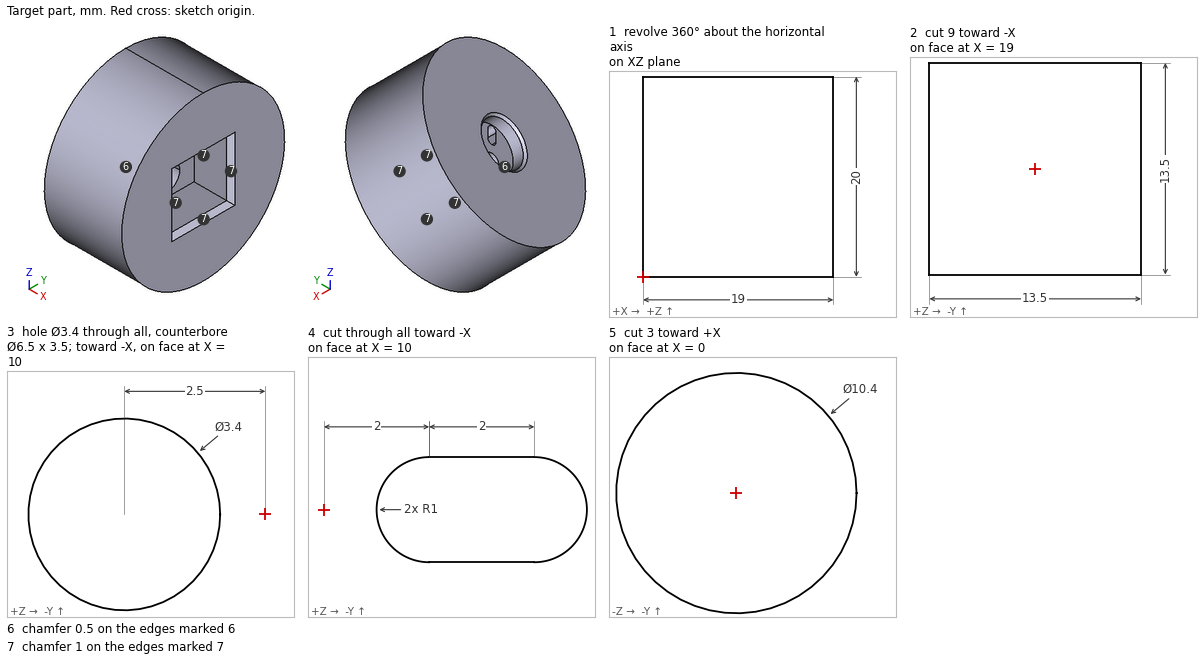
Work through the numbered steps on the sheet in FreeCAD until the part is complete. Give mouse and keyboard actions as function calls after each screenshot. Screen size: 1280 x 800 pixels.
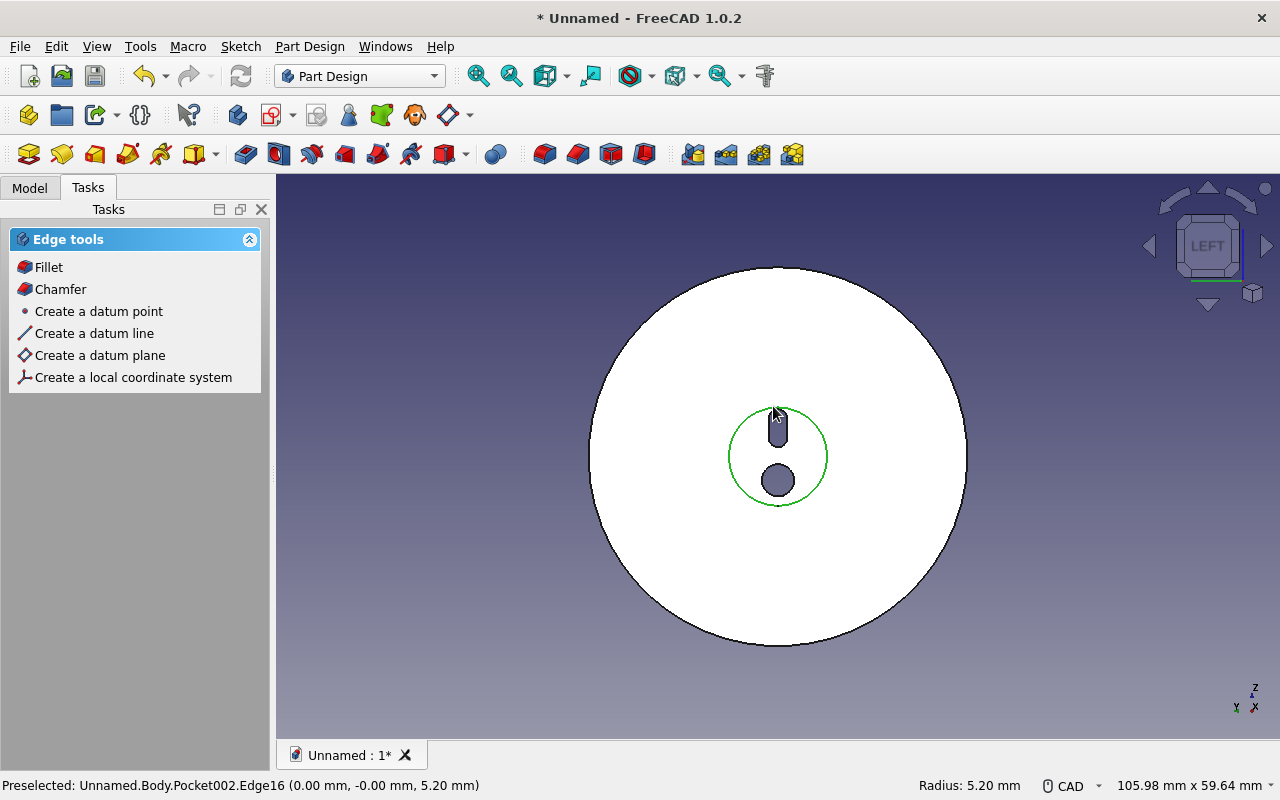
click(578, 154)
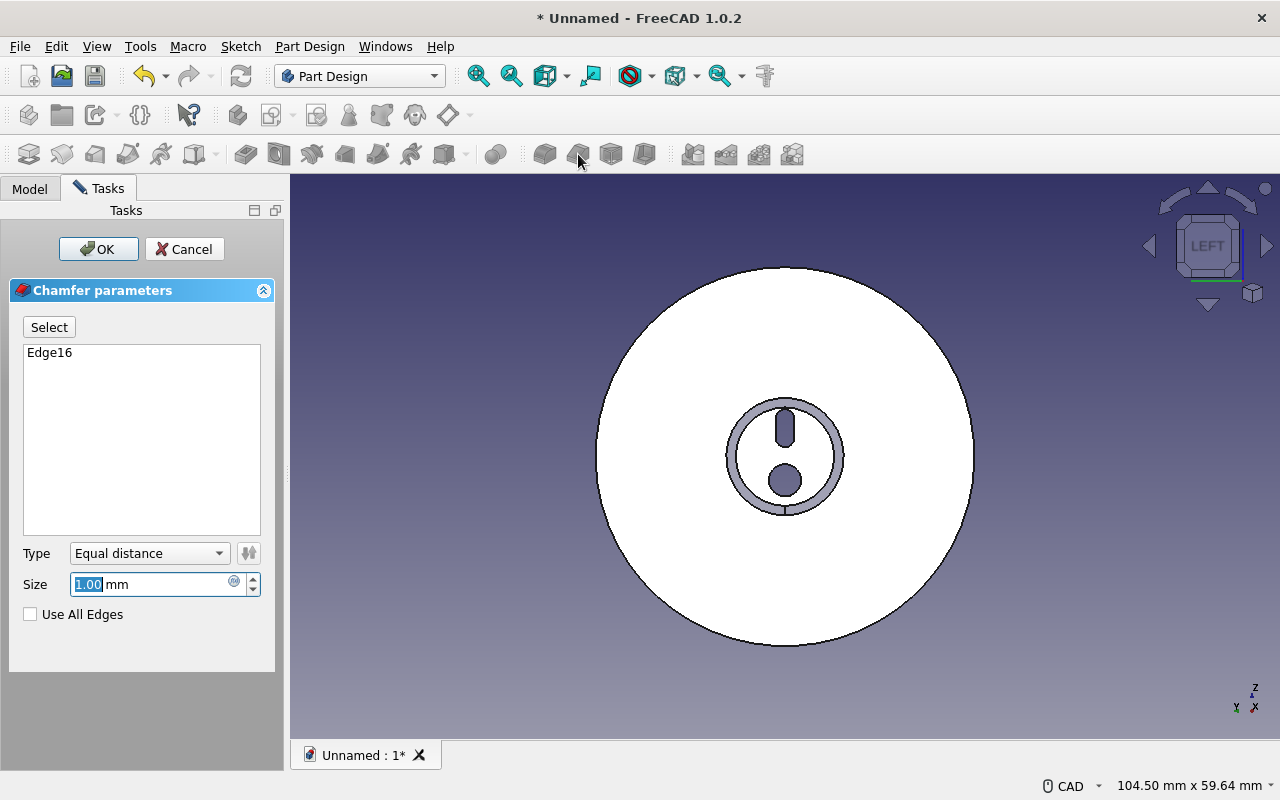
text(0.5)
key(Tab)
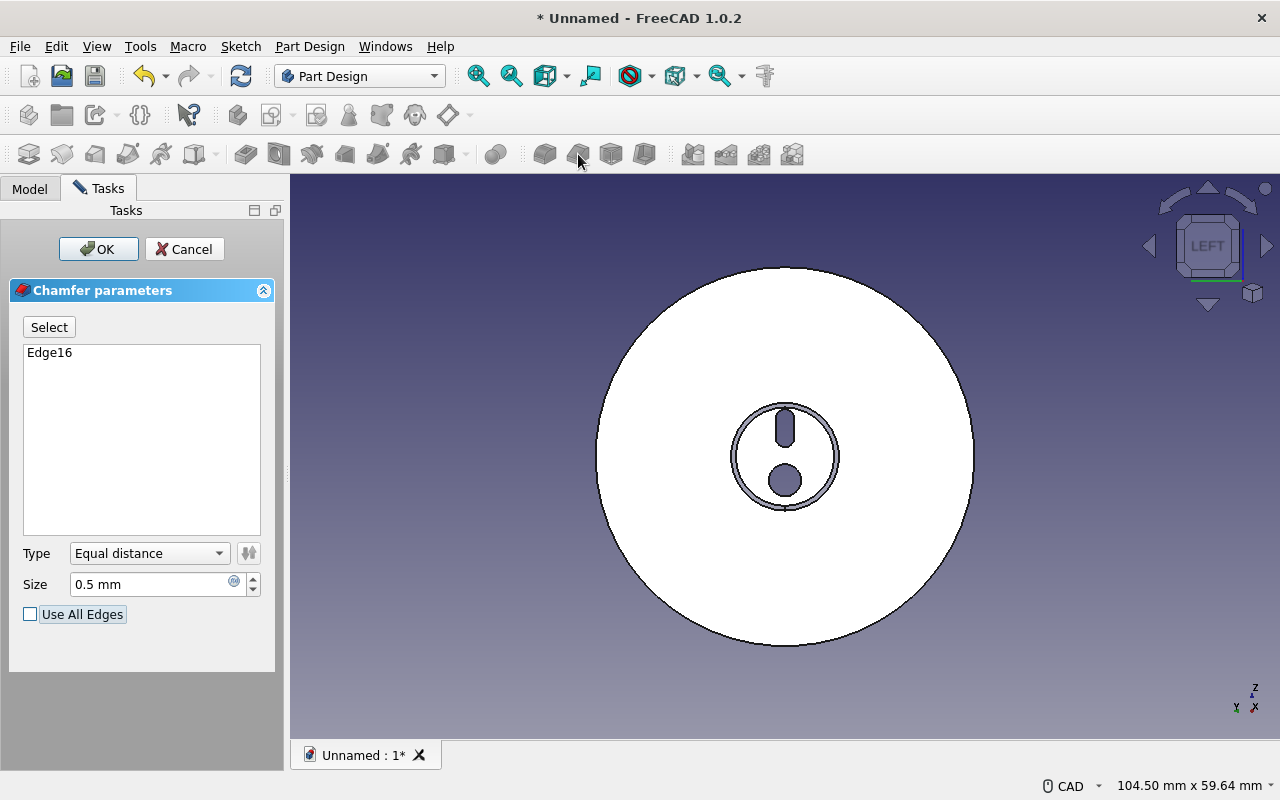
click(99, 249)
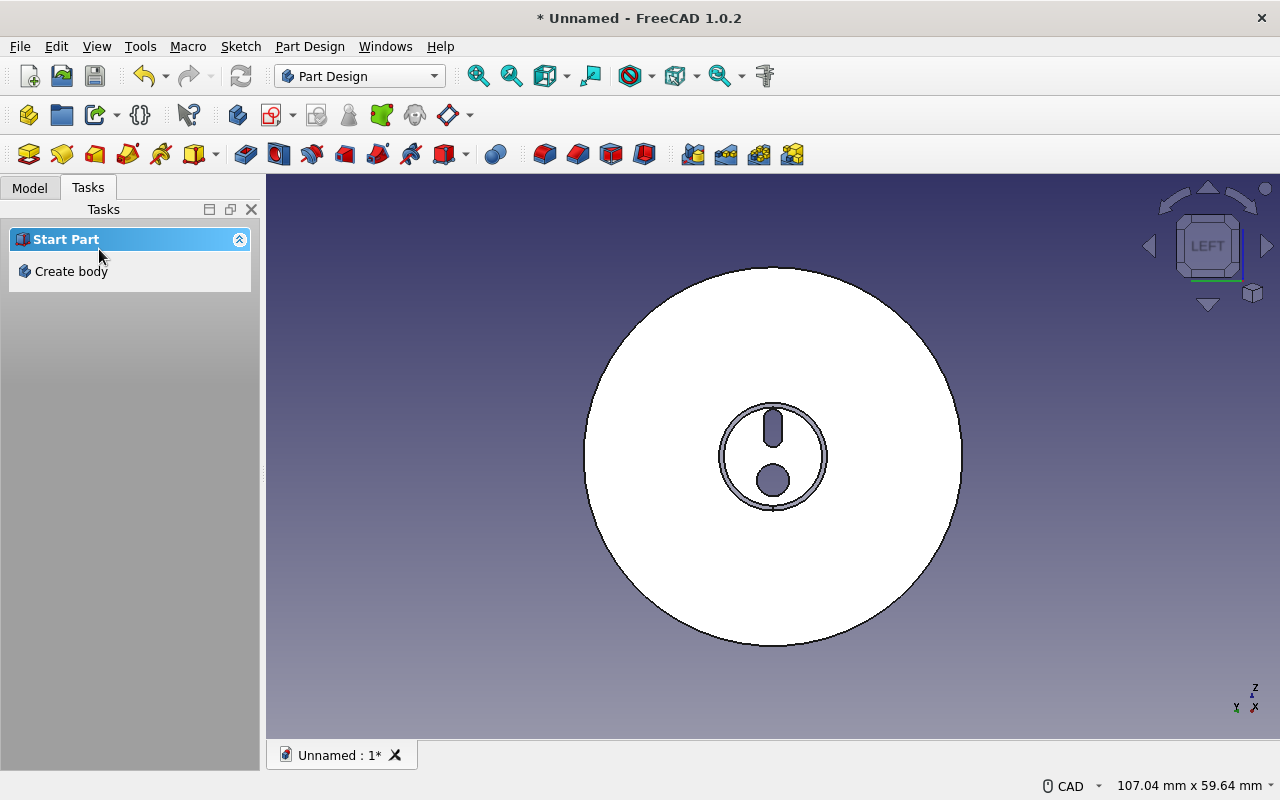
key(0)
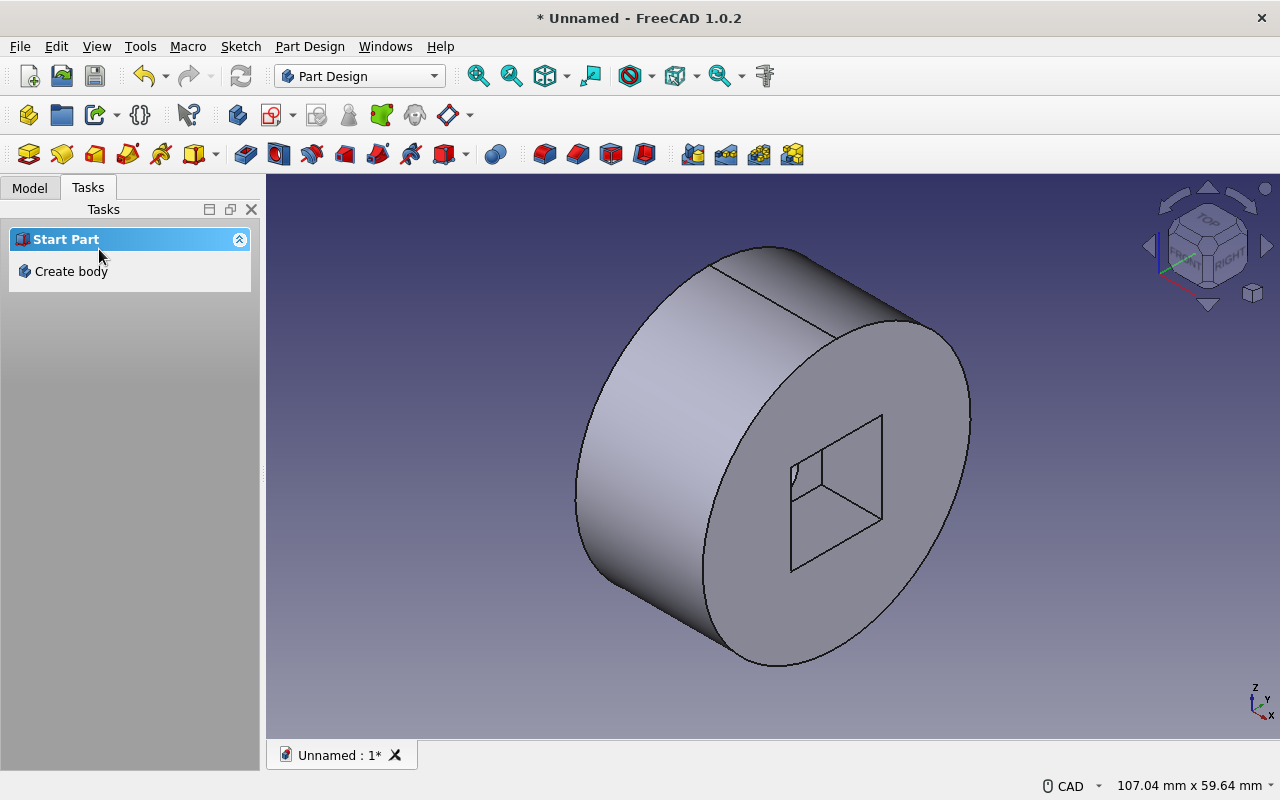
click(837, 545)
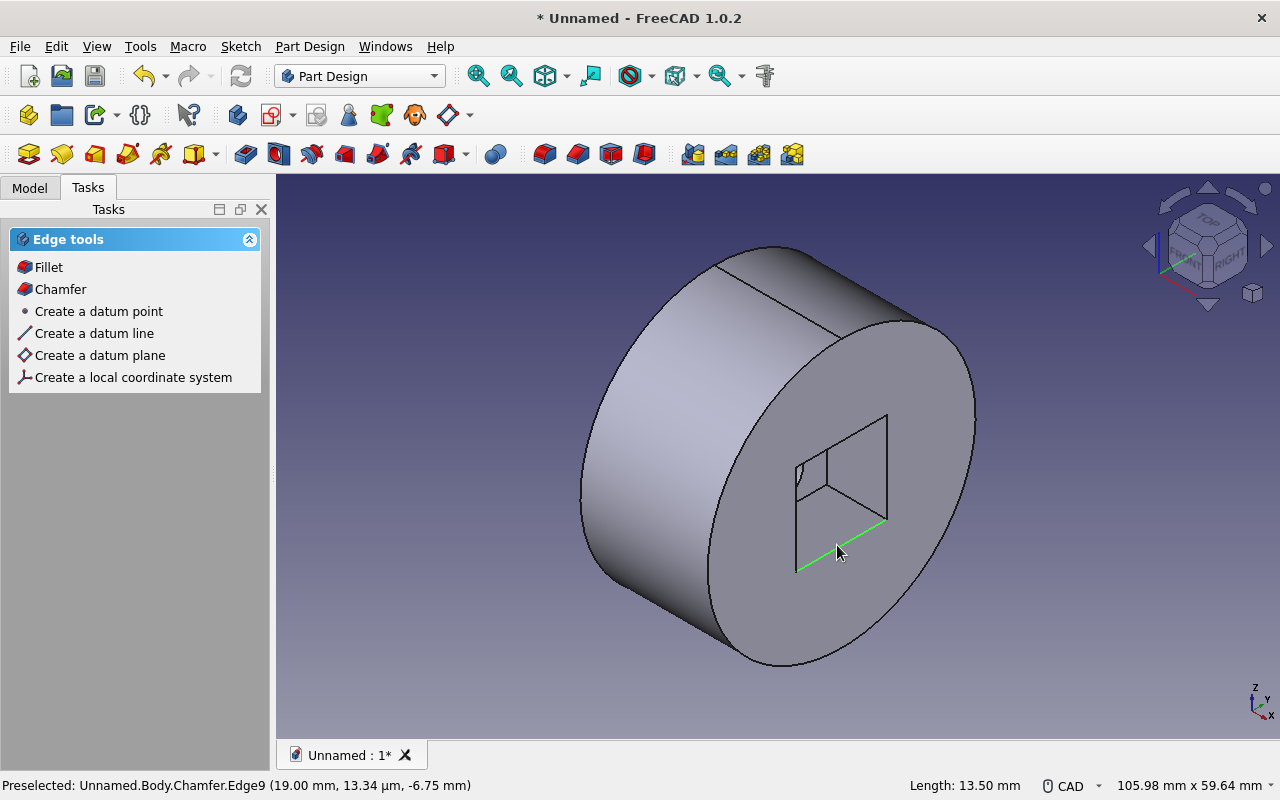
click(887, 466, ctrl)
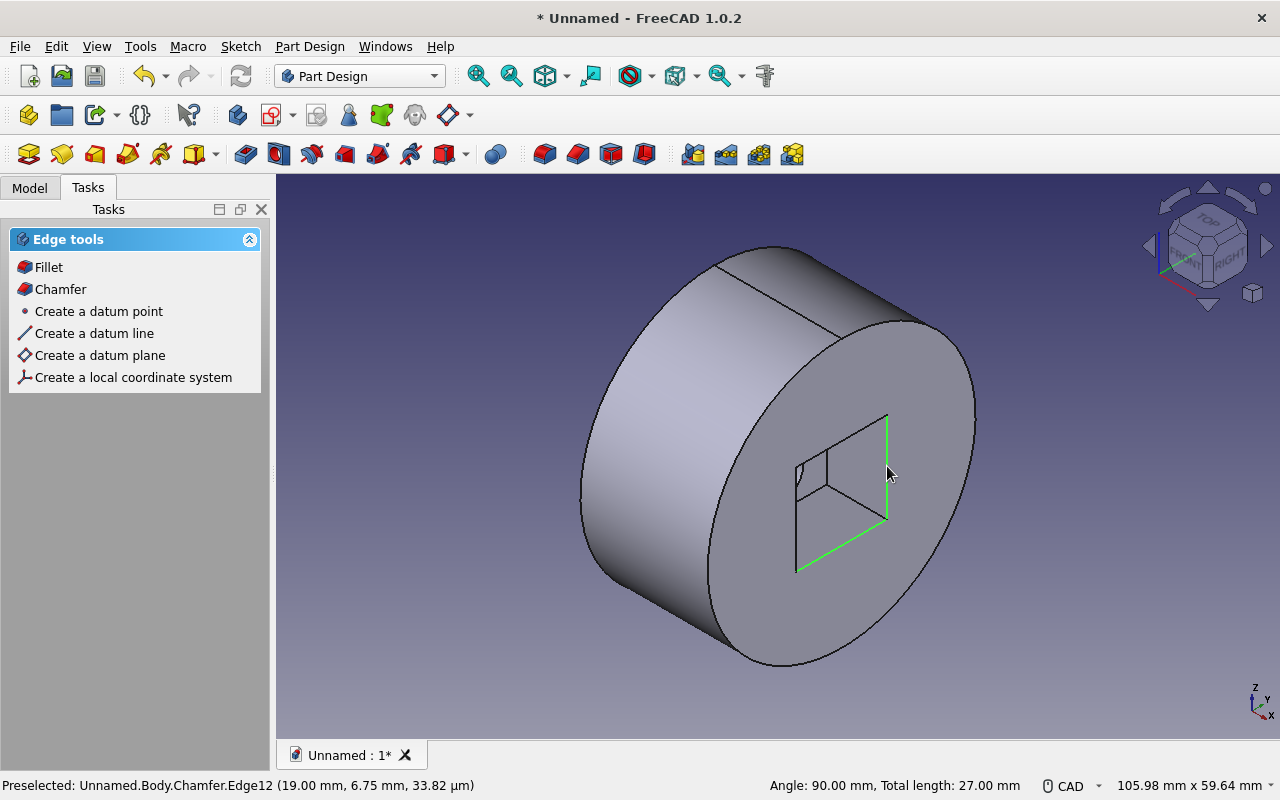
key(2)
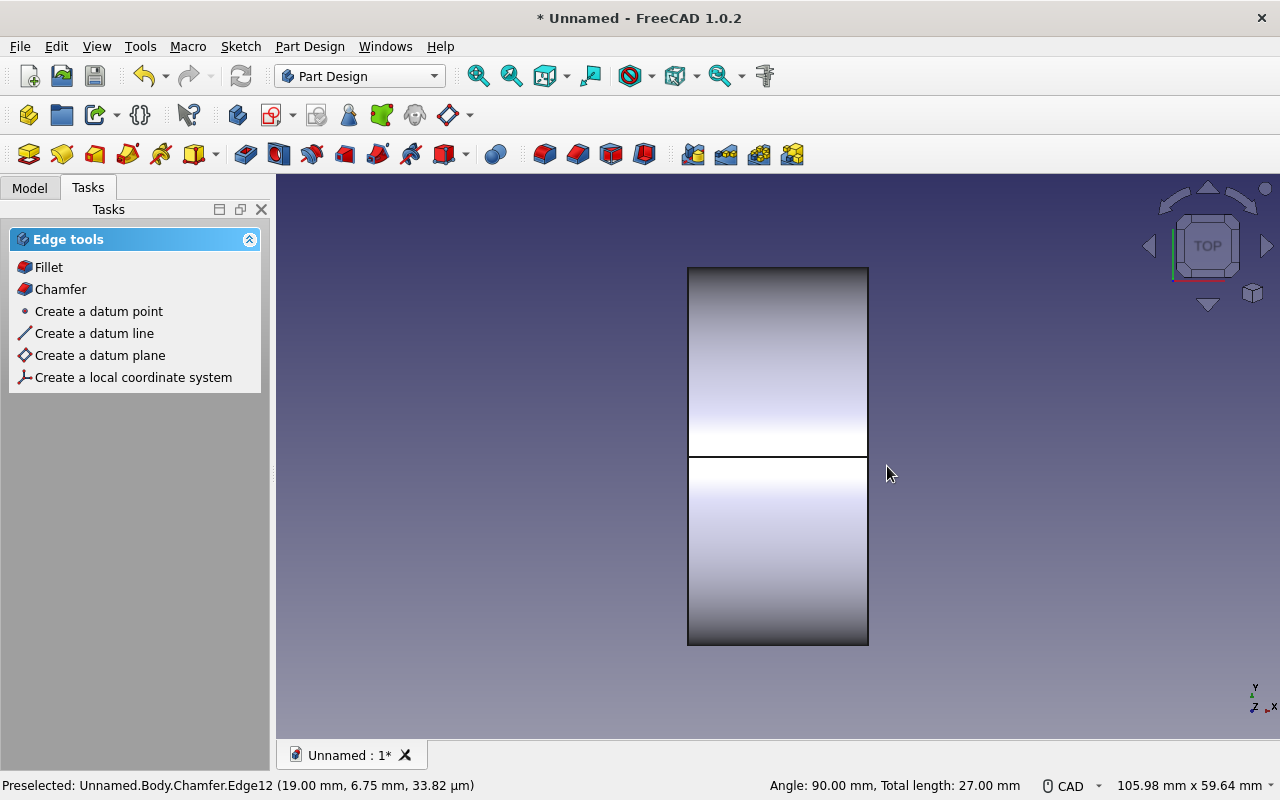
key(1)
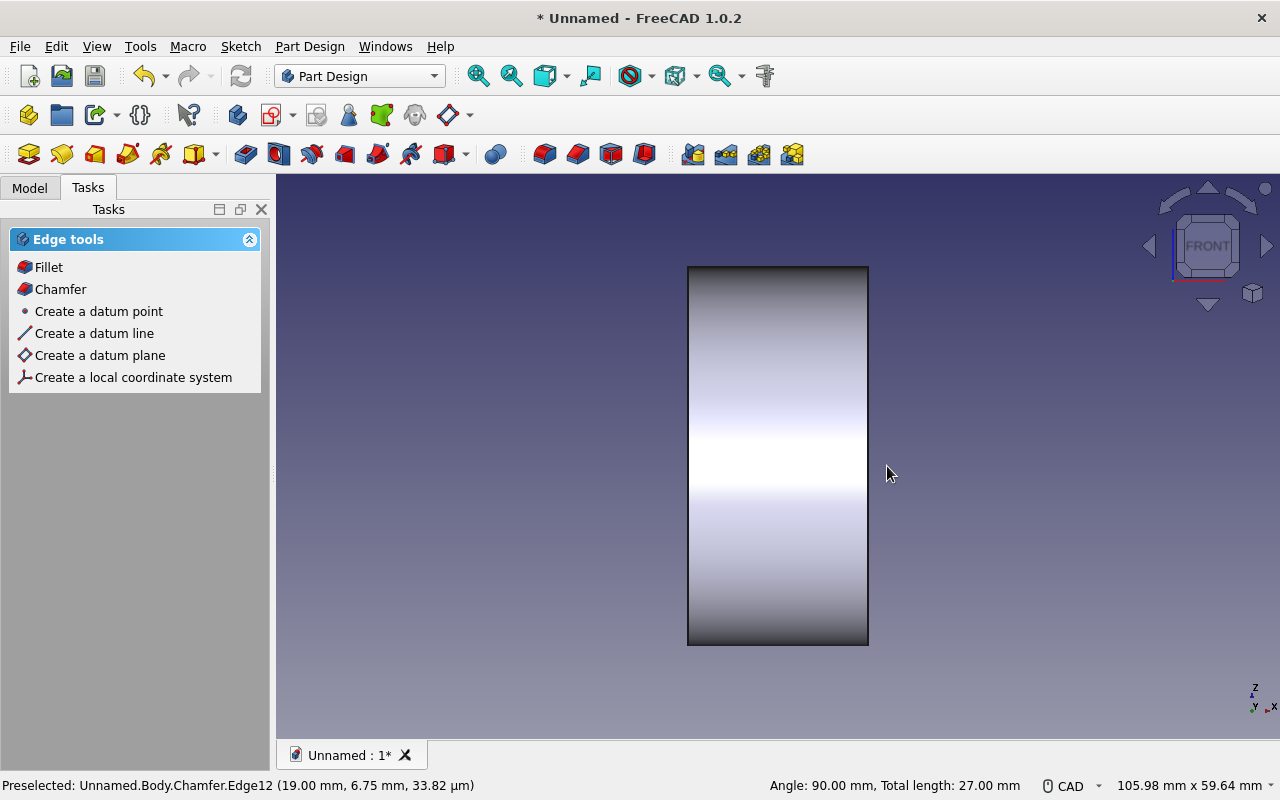
key(3)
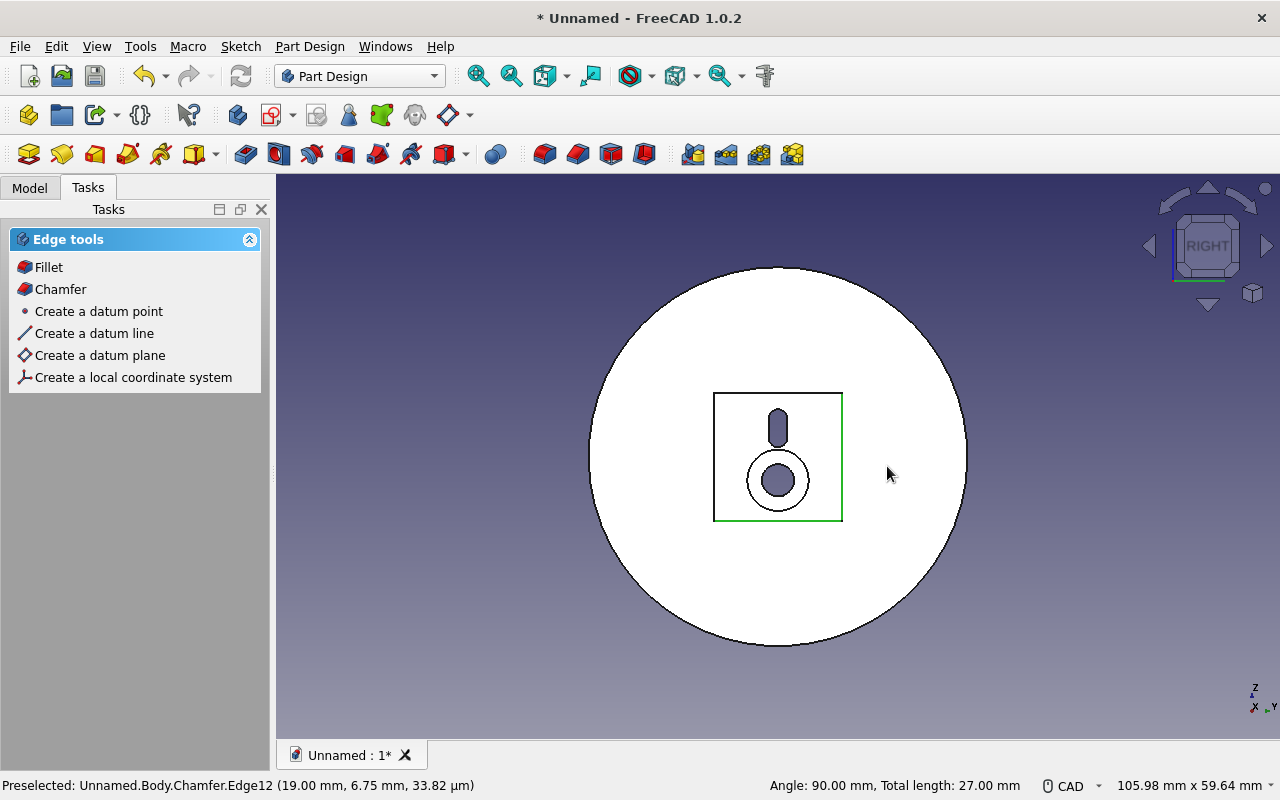
click(778, 392, ctrl)